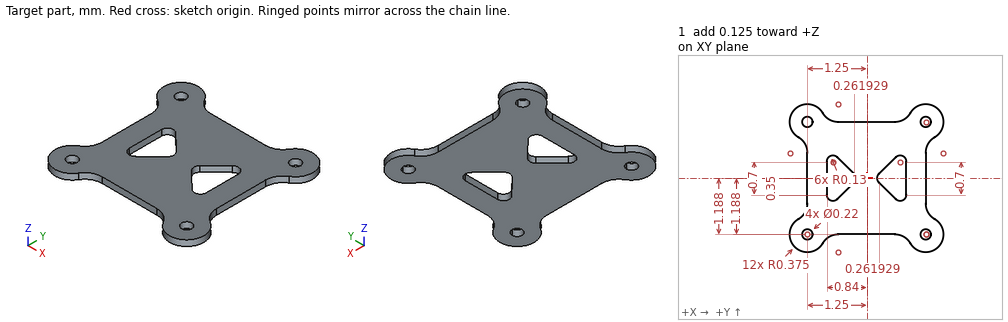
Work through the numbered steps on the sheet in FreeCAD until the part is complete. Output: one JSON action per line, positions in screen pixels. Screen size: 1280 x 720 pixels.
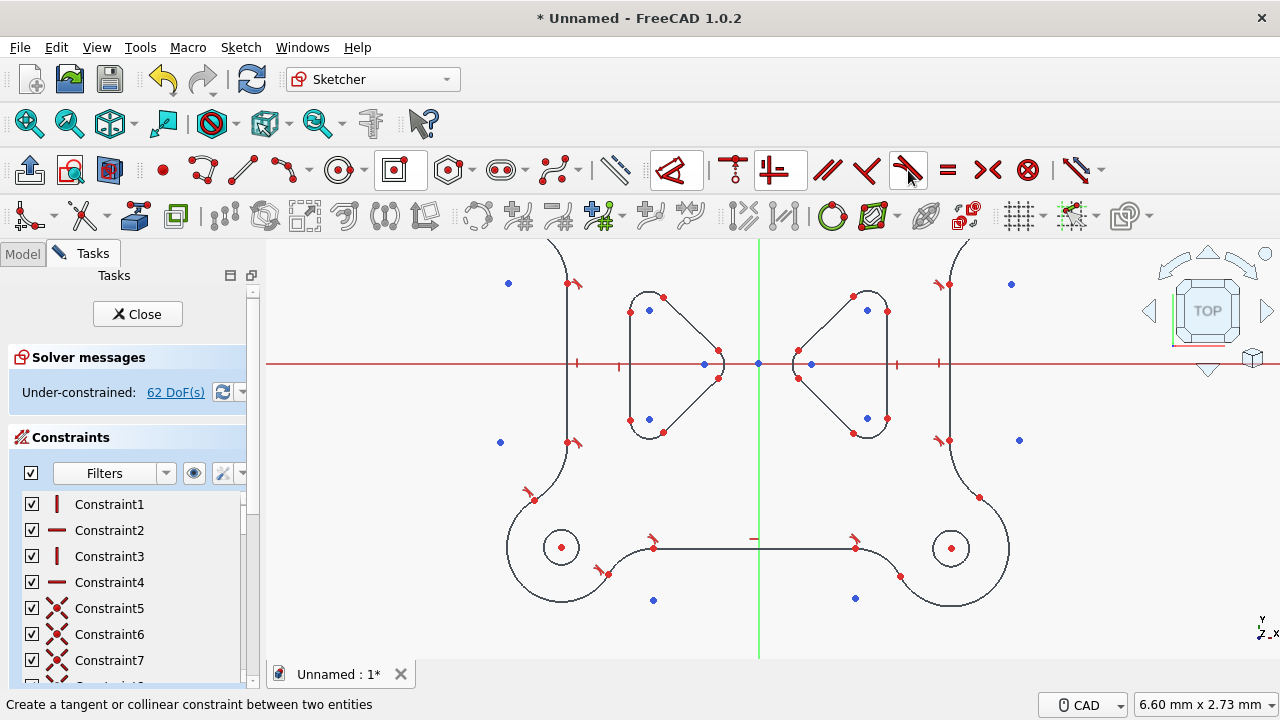
{"action": "left_click", "coordinate": [891, 563]}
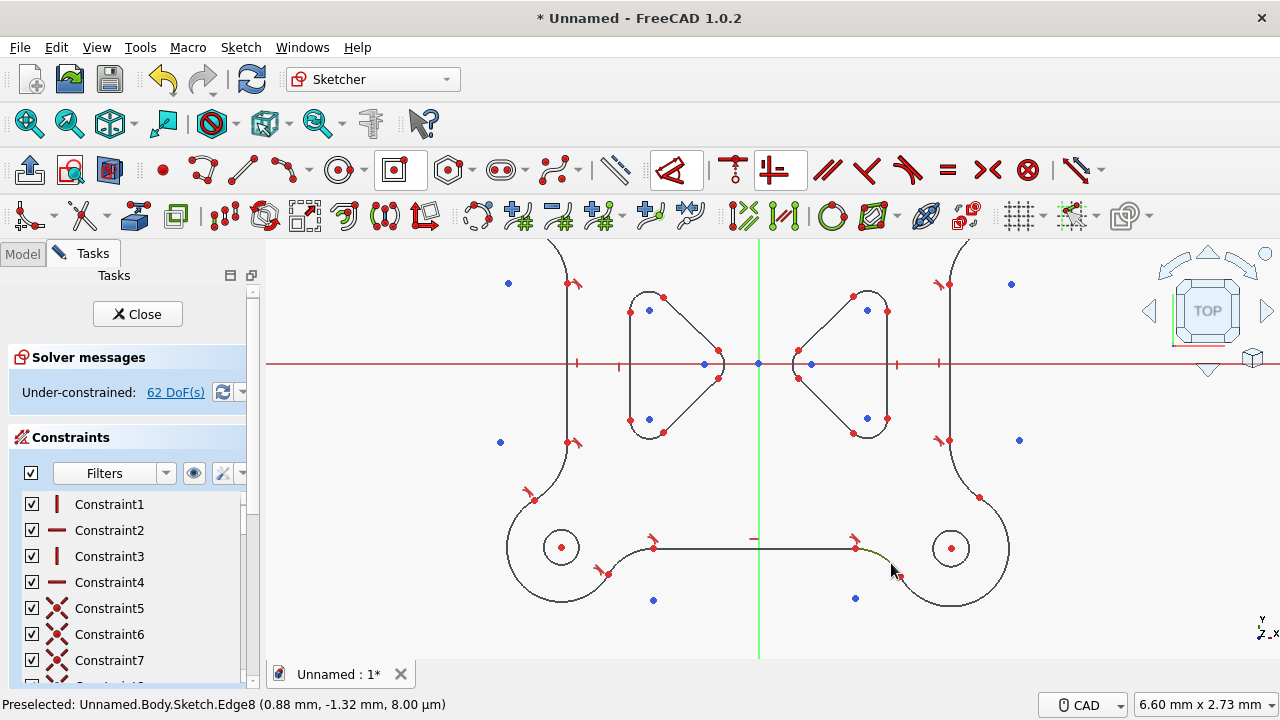
{"action": "left_click", "coordinate": [954, 606]}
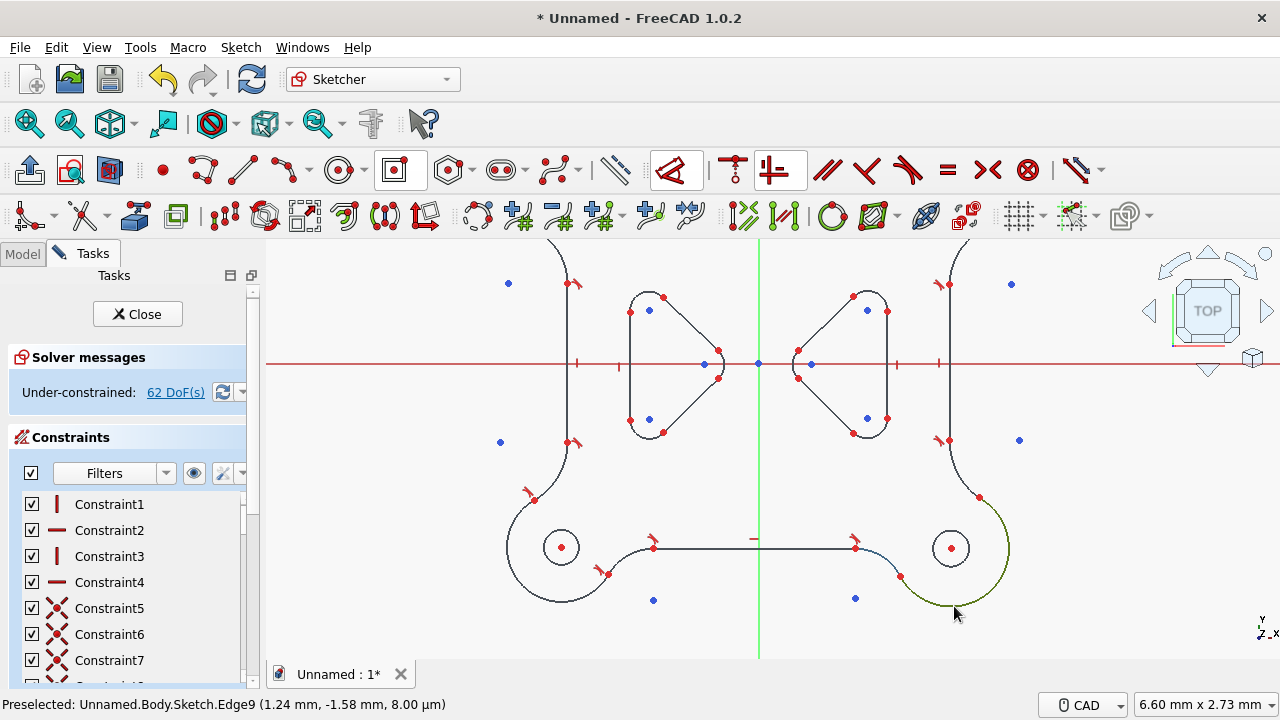
{"action": "left_click", "coordinate": [908, 170]}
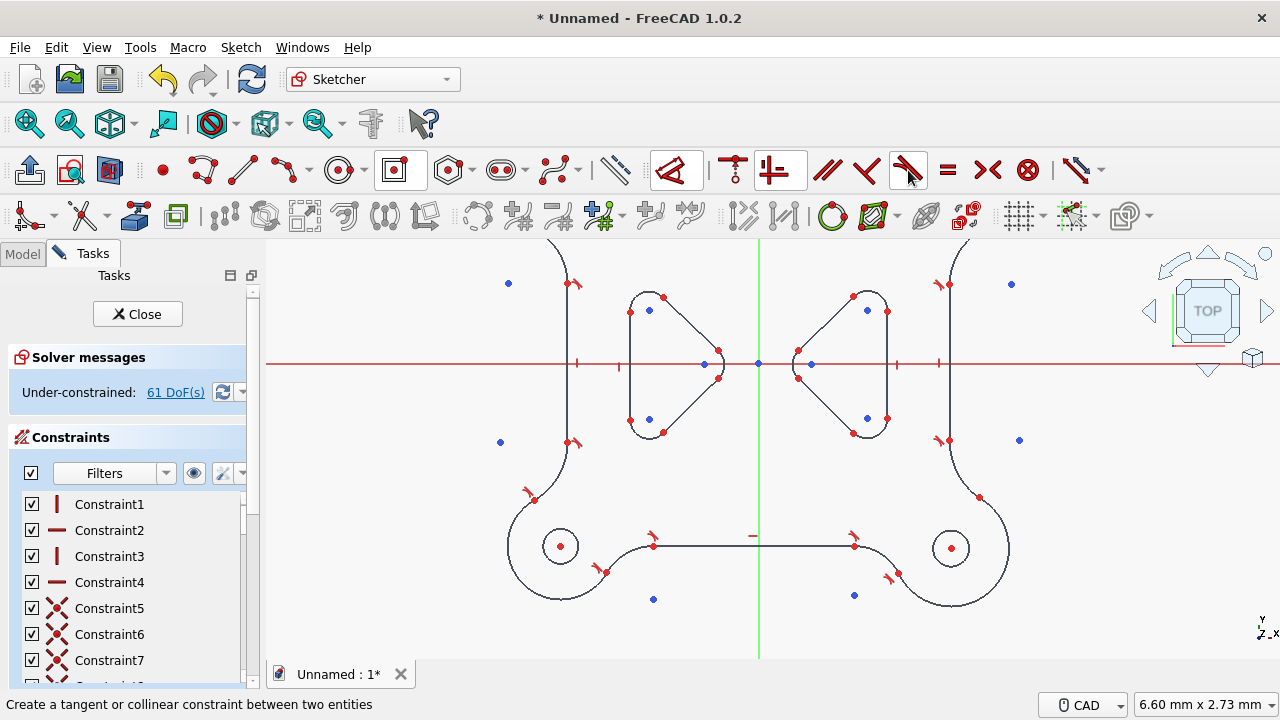
{"action": "left_click", "coordinate": [952, 607]}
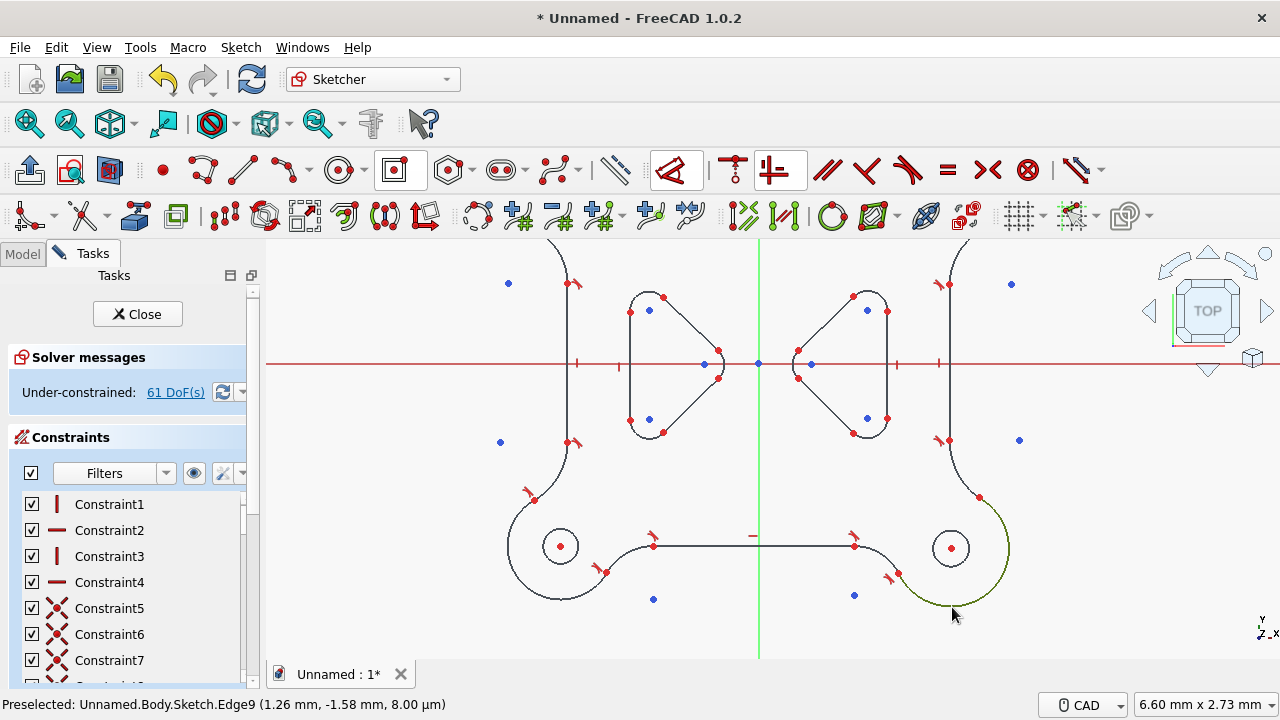
{"action": "left_click", "coordinate": [953, 461]}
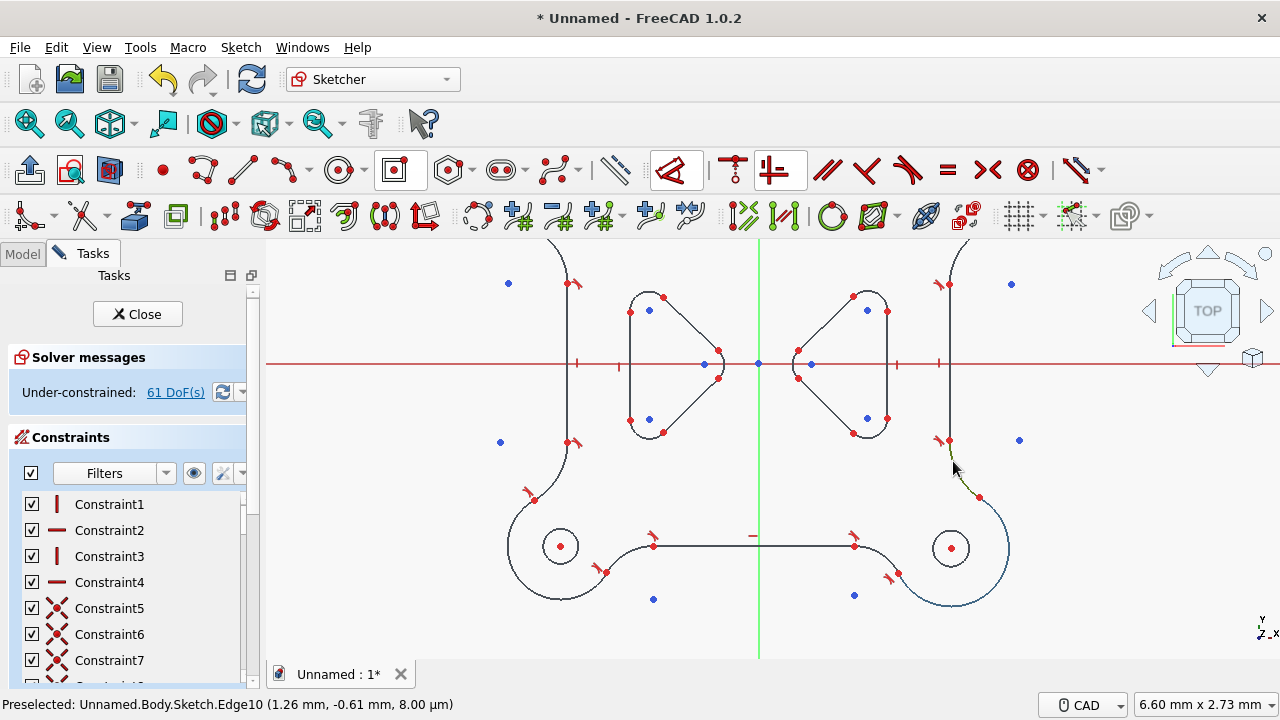
{"action": "left_click", "coordinate": [908, 170]}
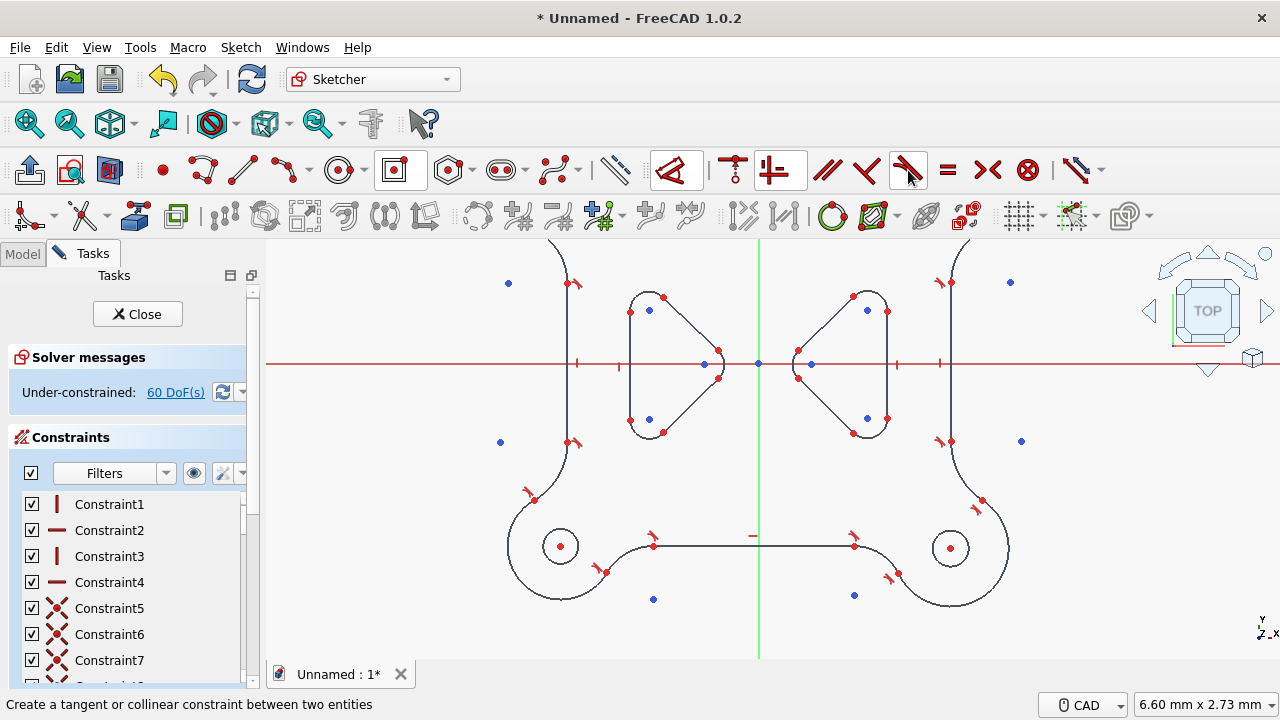
{"action": "left_click", "coordinate": [952, 271]}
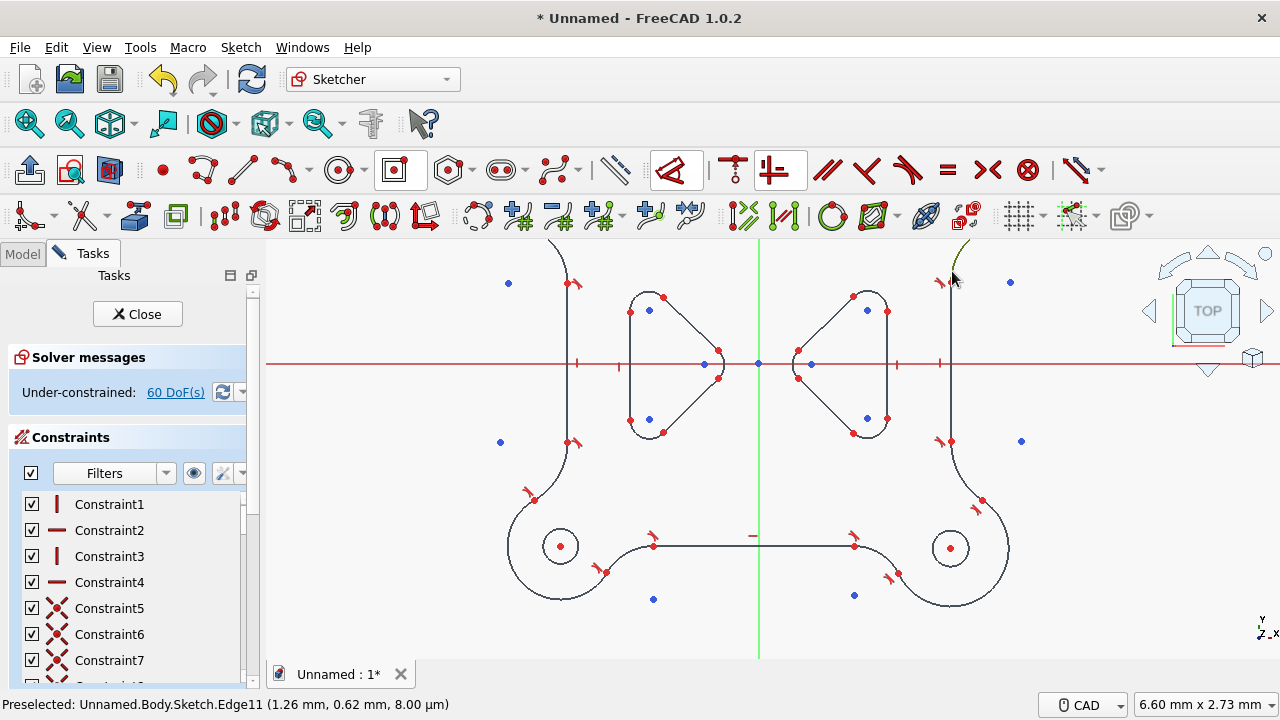
{"action": "scroll", "coordinate": [639, 552], "scroll_direction": "down", "scroll_amount": 3}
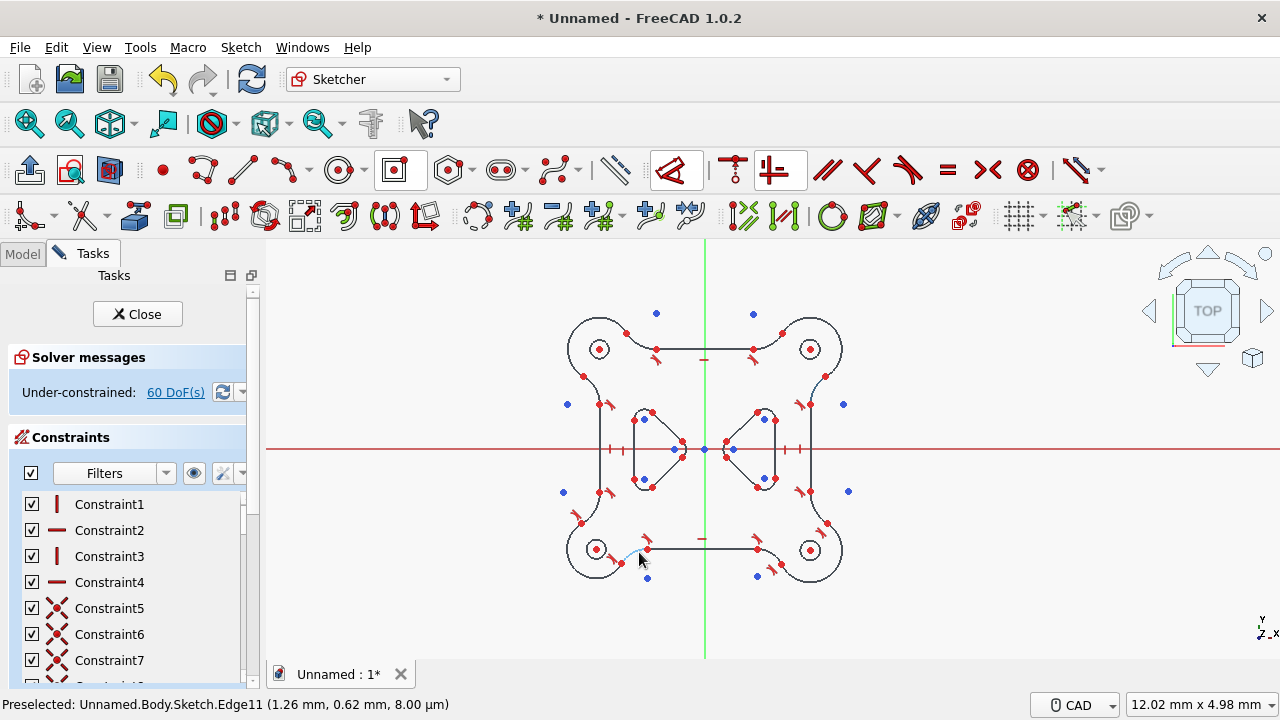
{"action": "left_click", "coordinate": [842, 348]}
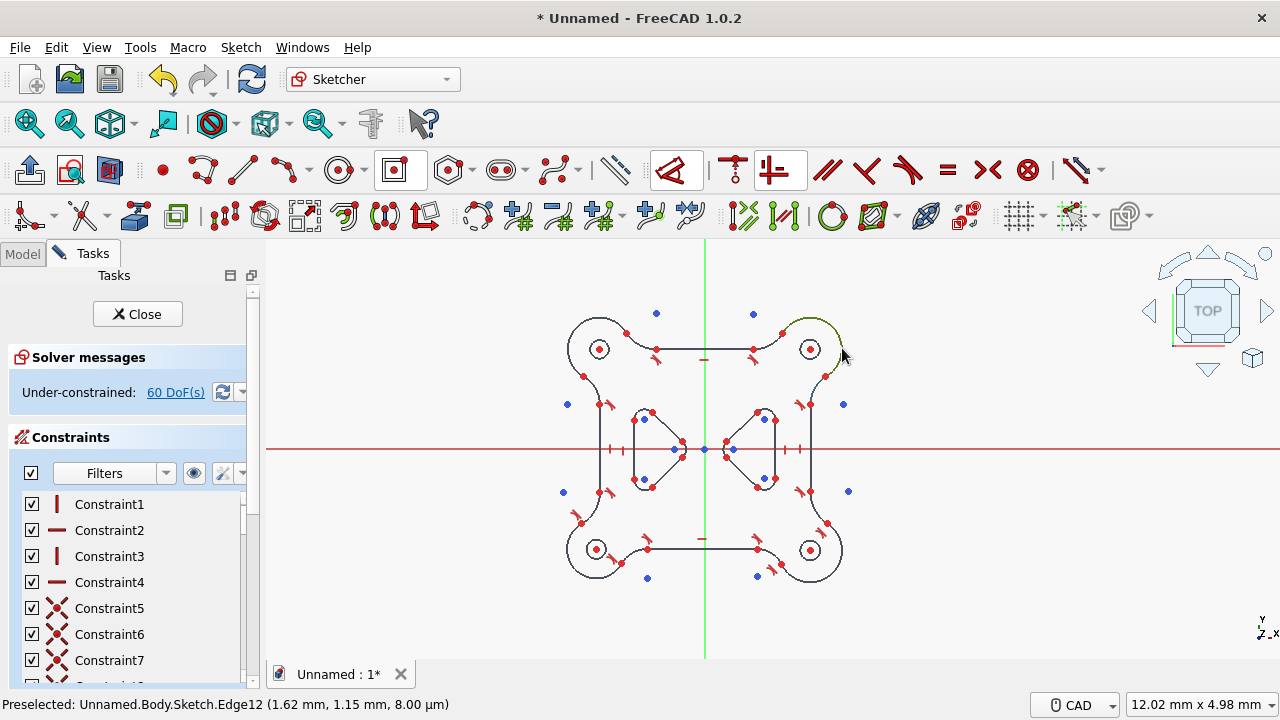
{"action": "left_click", "coordinate": [908, 170]}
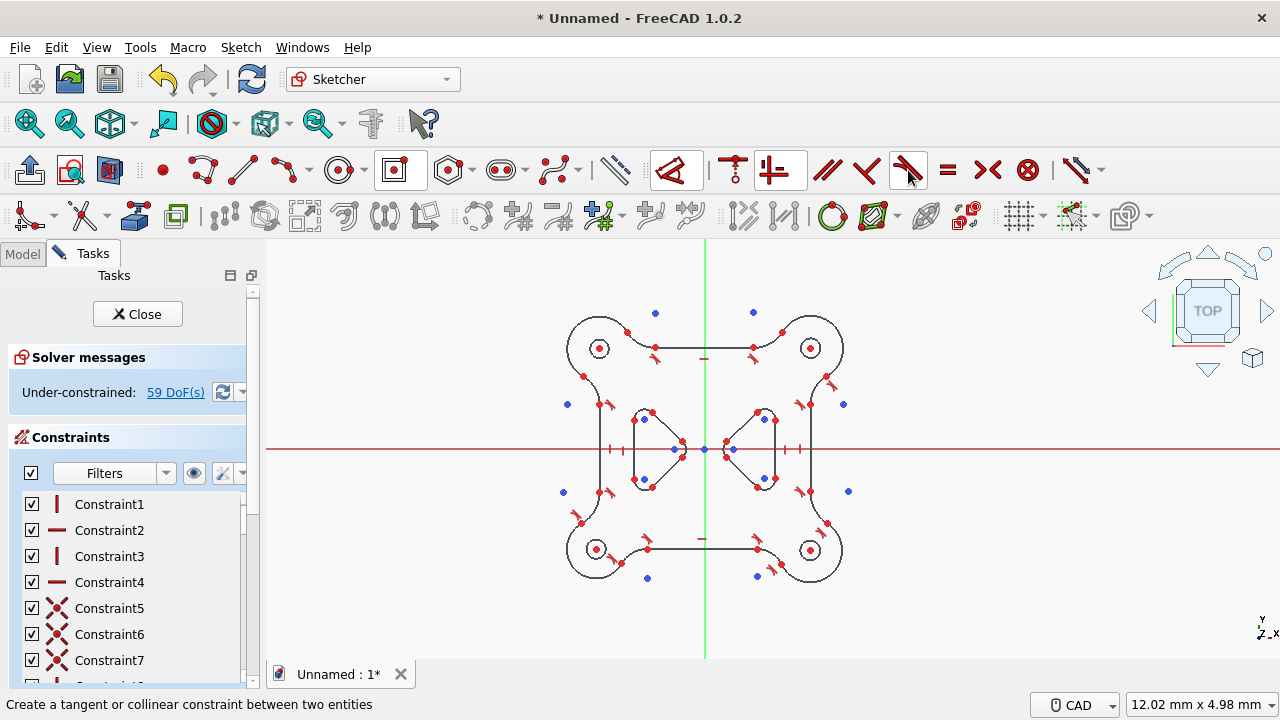
{"action": "left_click", "coordinate": [843, 346]}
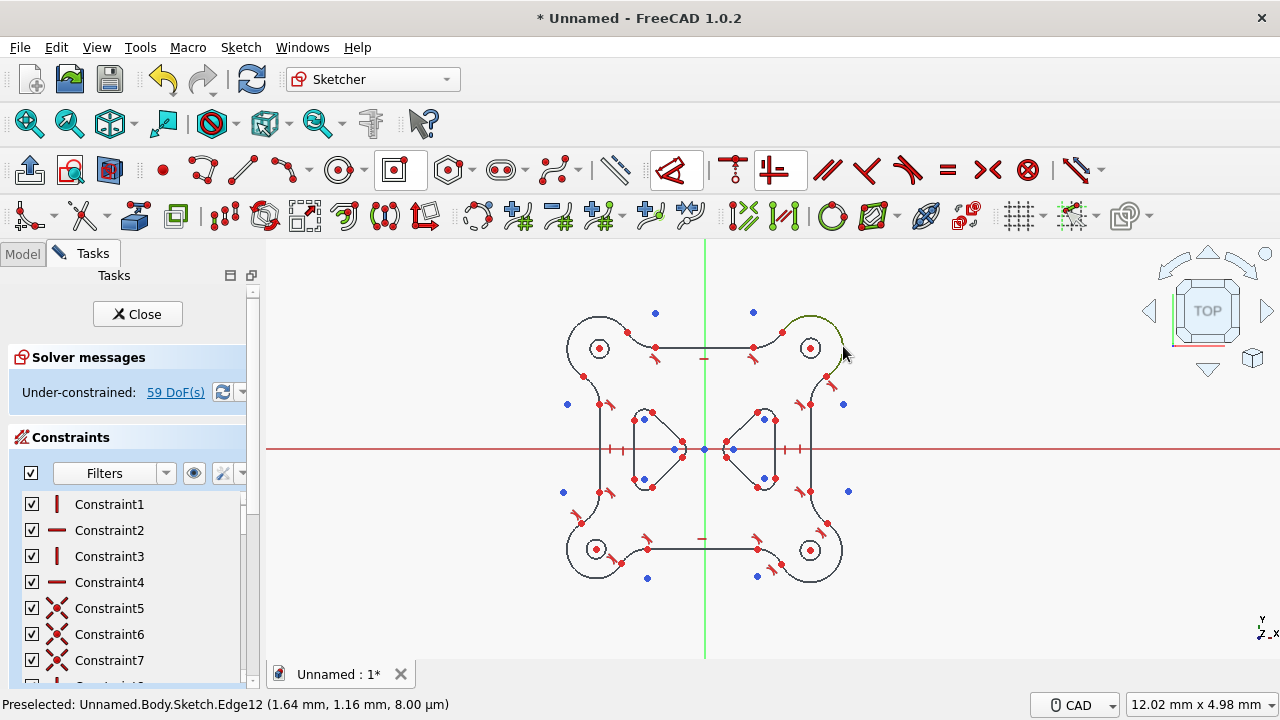
{"action": "scroll", "coordinate": [764, 346], "scroll_direction": "up", "scroll_amount": 2}